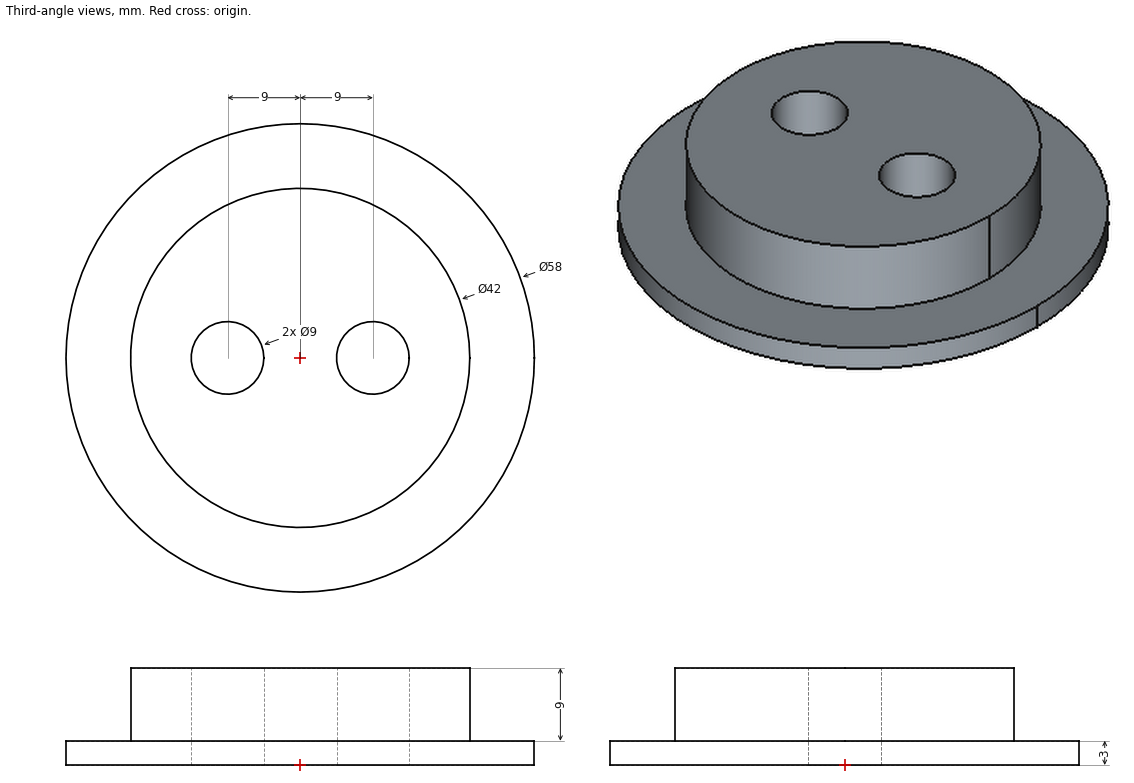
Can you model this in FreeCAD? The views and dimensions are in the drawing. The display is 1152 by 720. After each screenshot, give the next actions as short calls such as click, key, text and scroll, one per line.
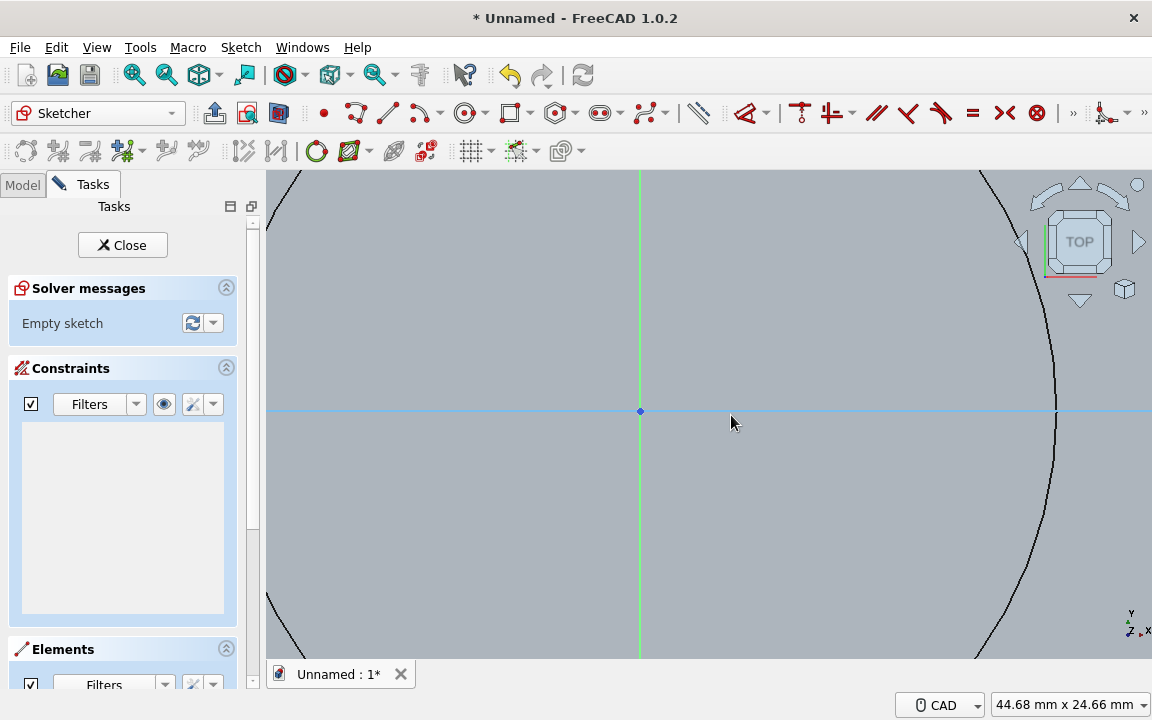
click(466, 114)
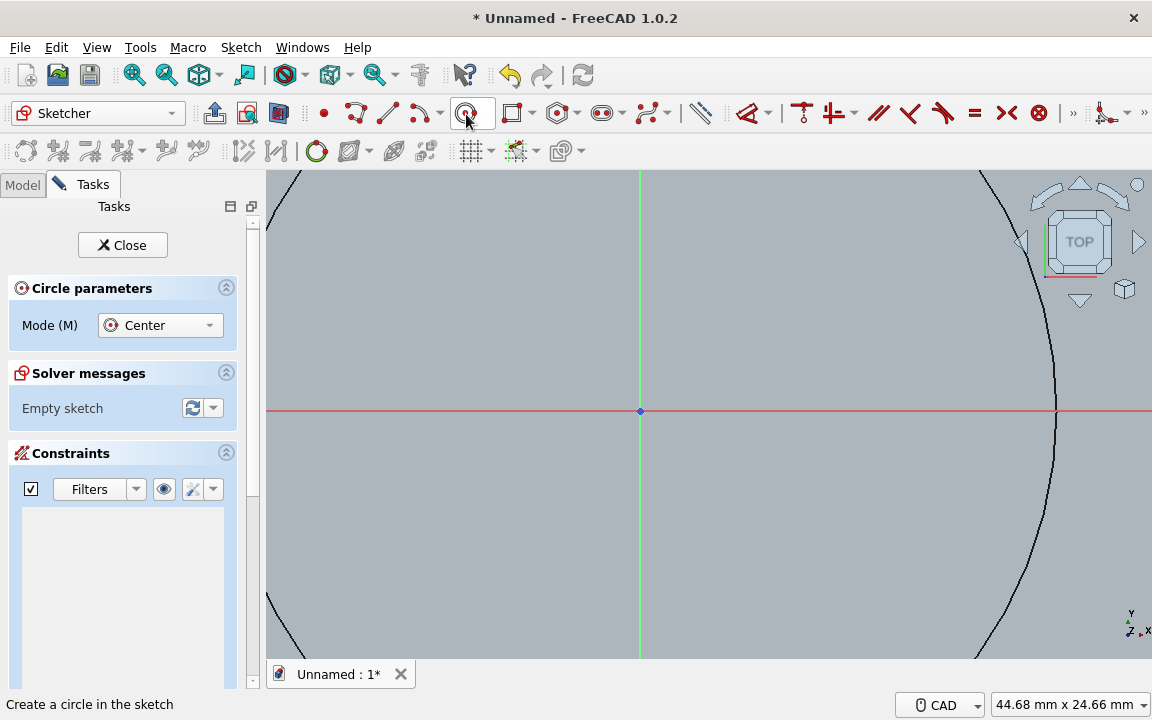
click(462, 411)
move(525, 348)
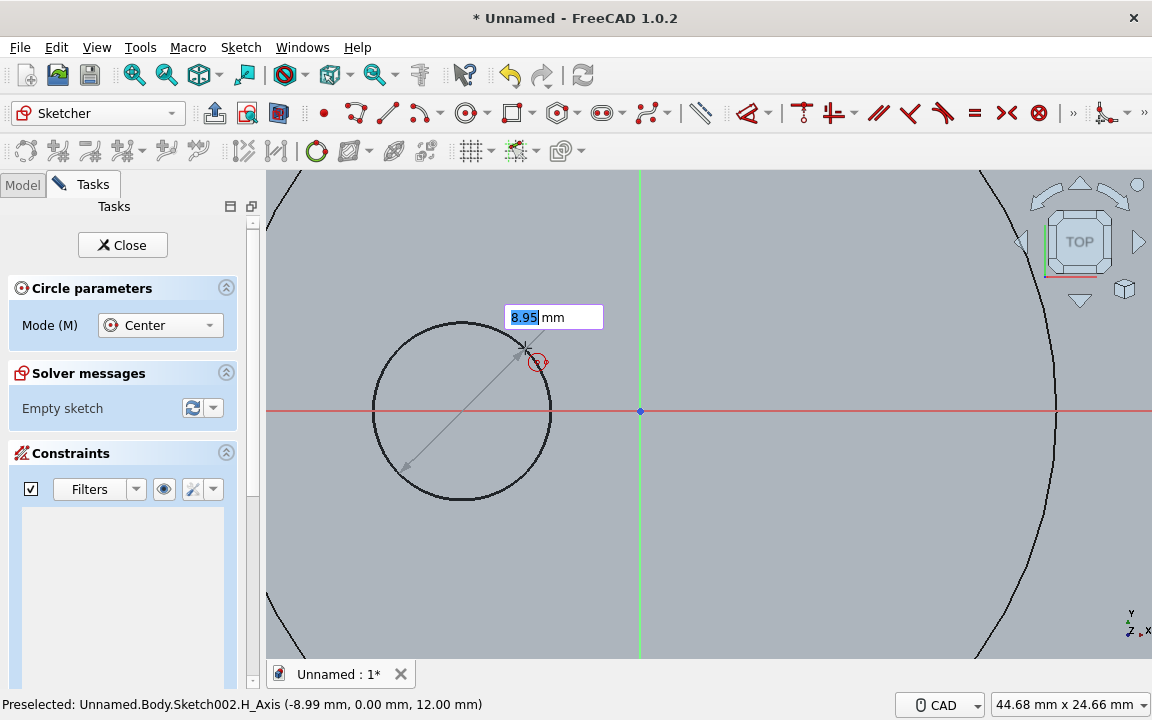
text(9)
key(Return)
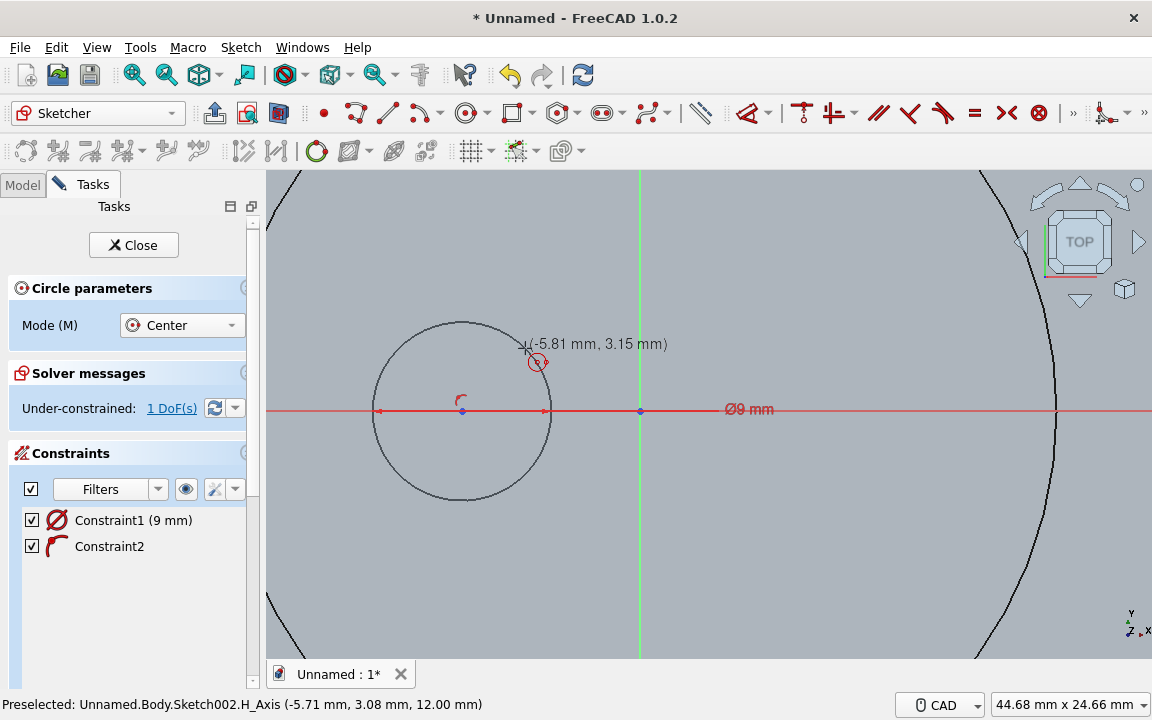
click(819, 411)
move(882, 348)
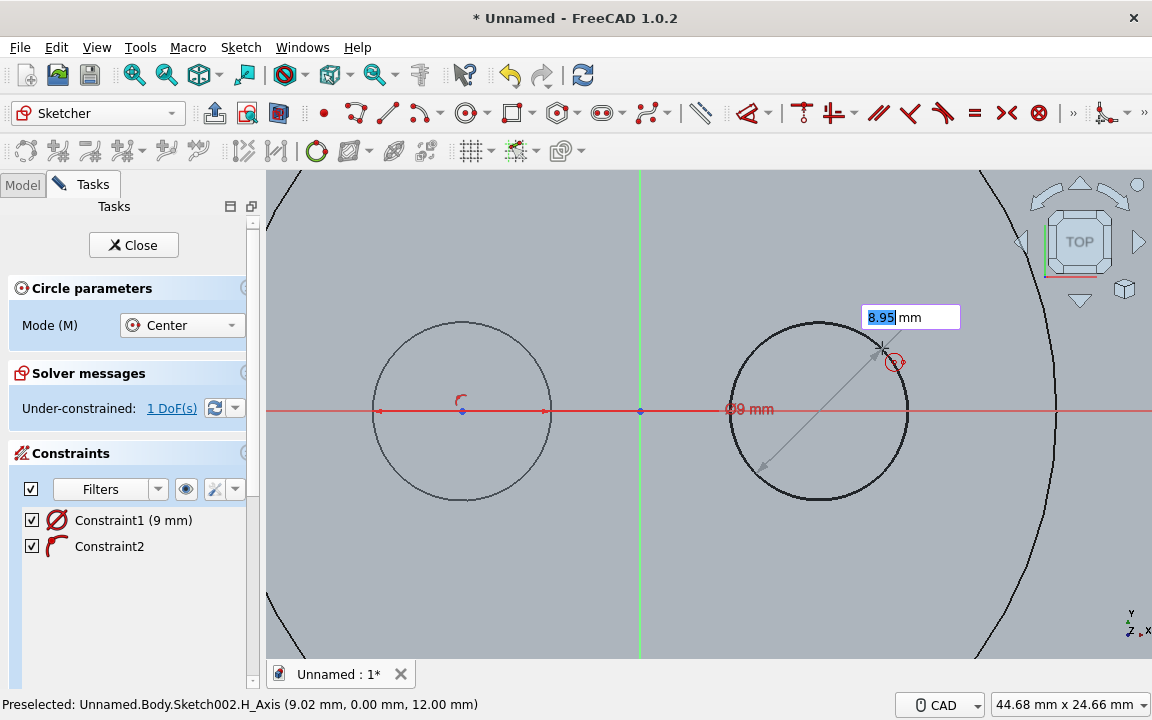
text(9)
key(Return)
key(Escape)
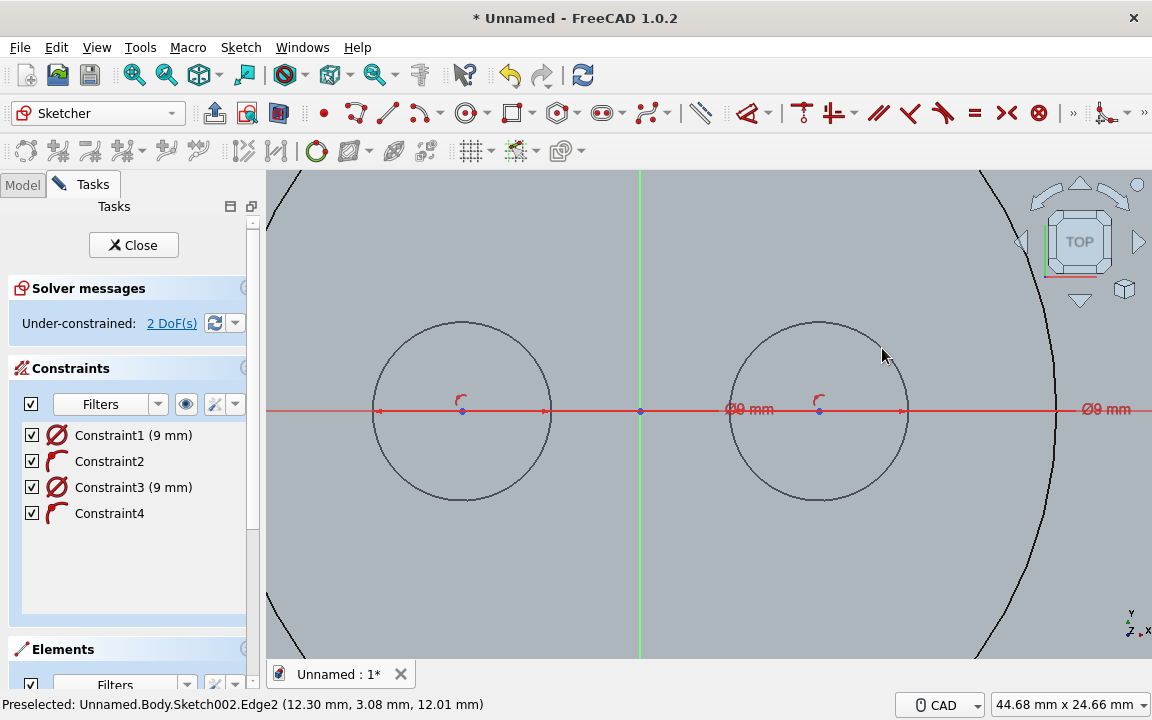
click(748, 114)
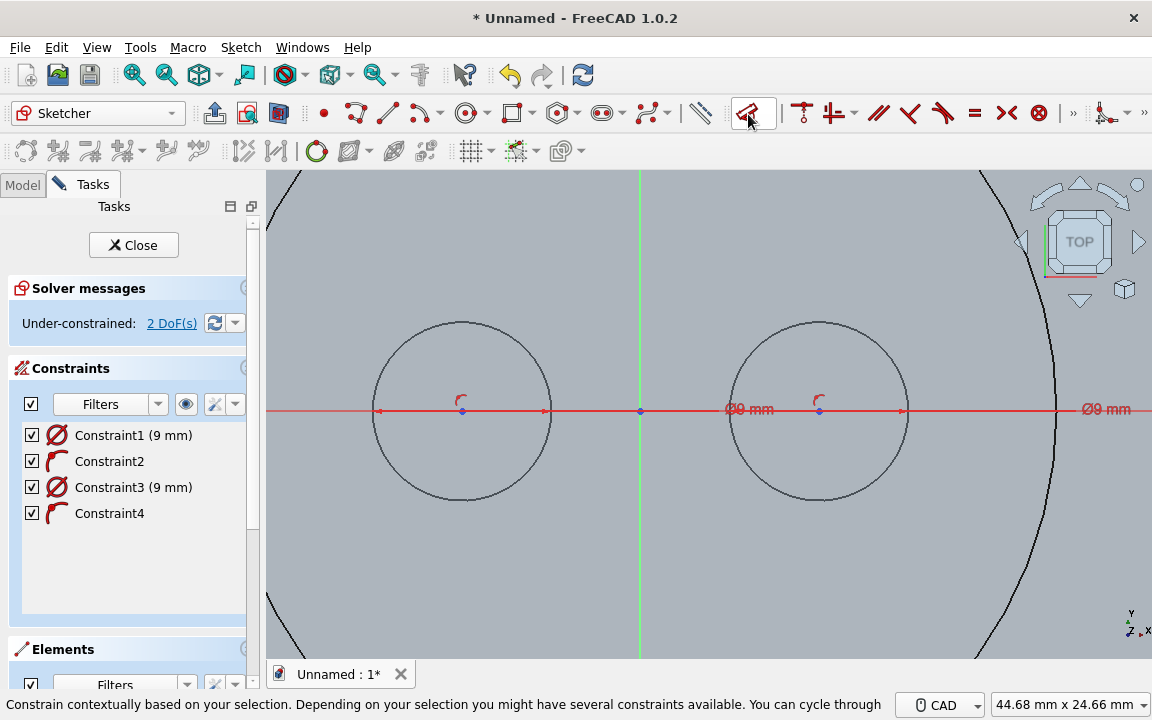
click(462, 411)
click(510, 445)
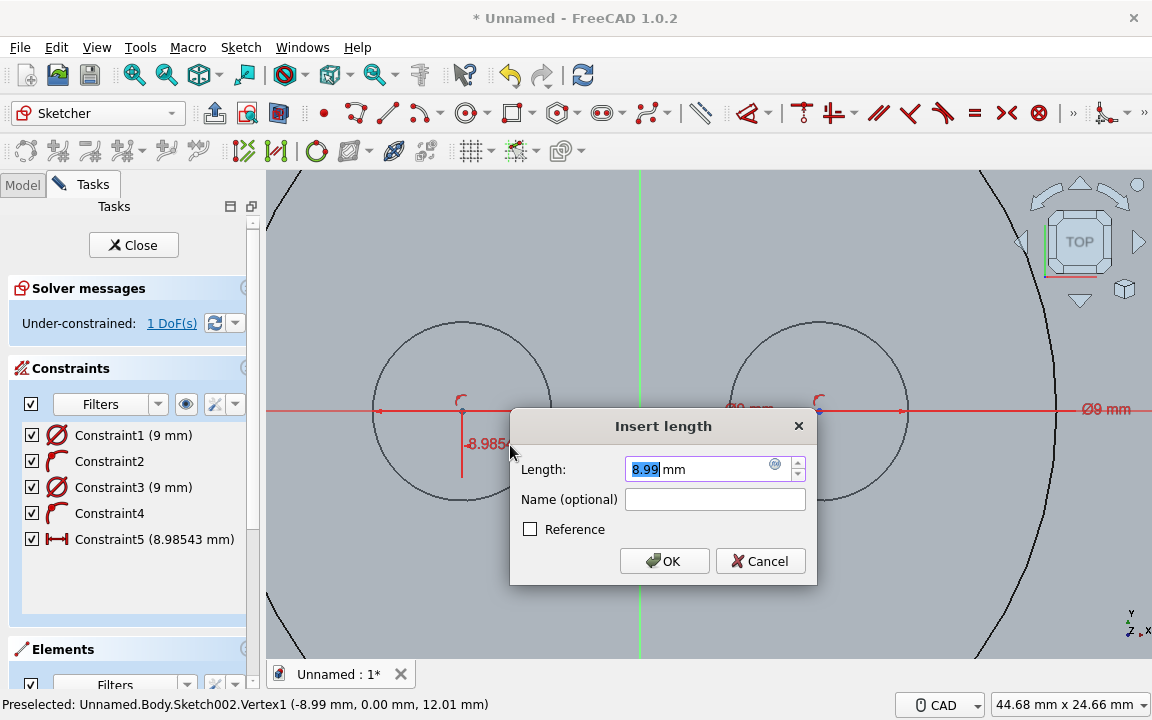
text(9)
key(Return)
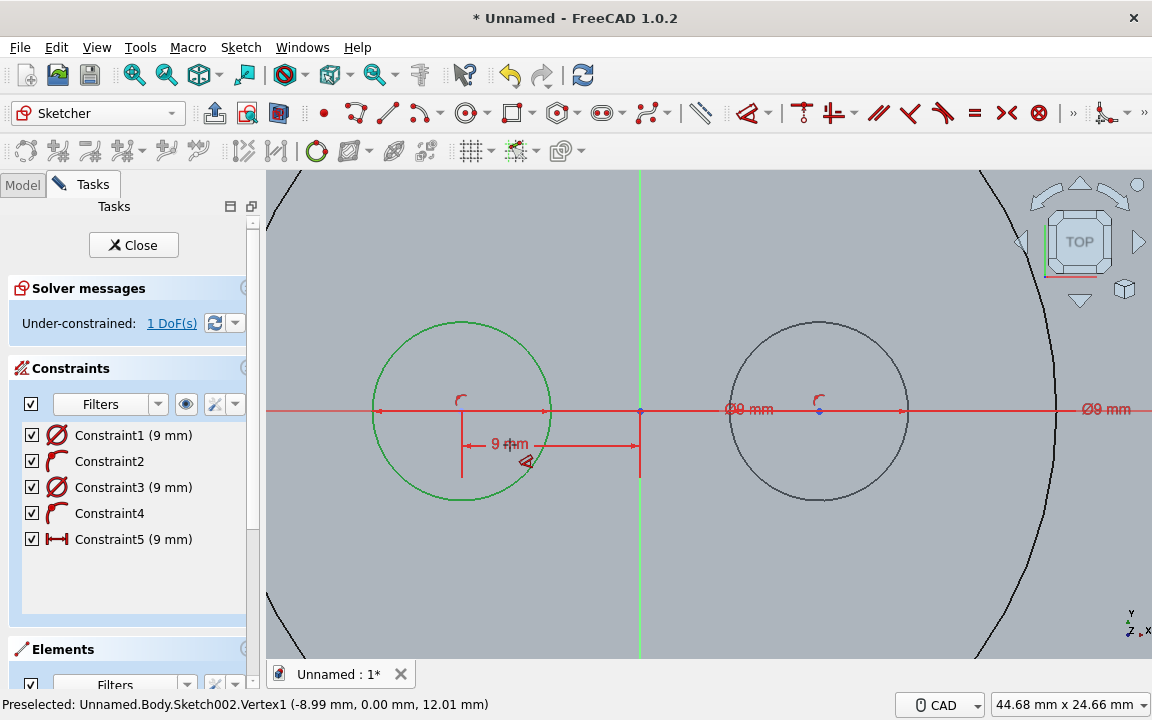
click(819, 411)
click(688, 445)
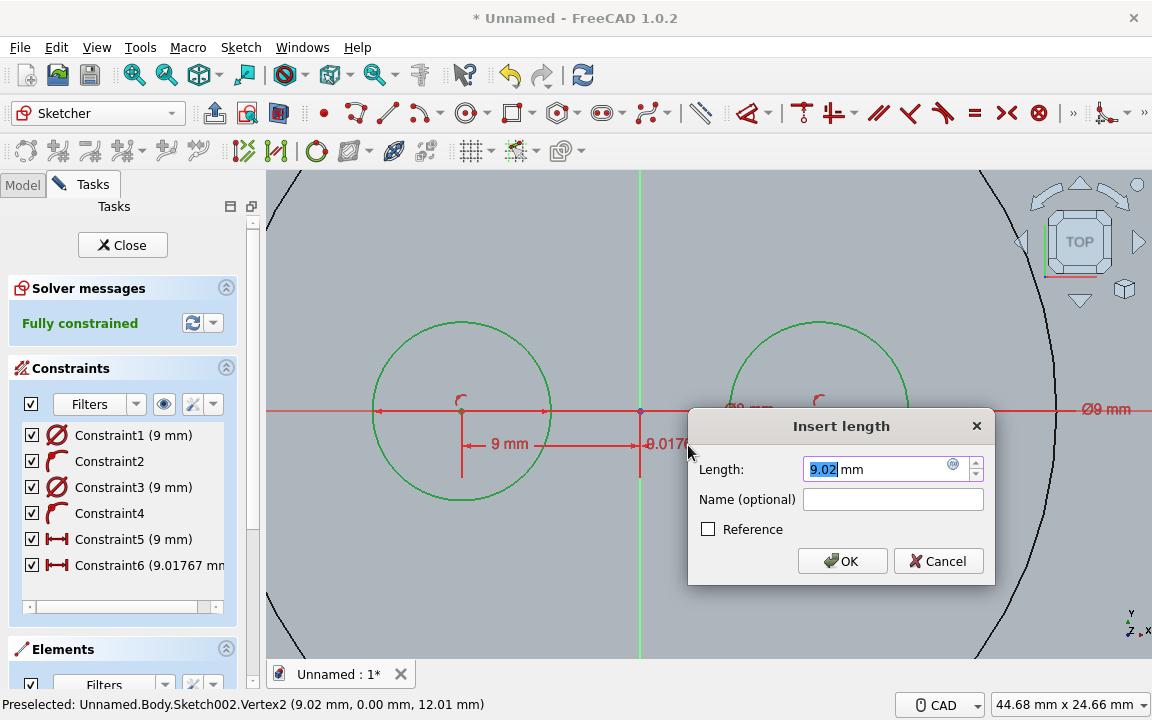
text(9)
key(Return)
key(Escape)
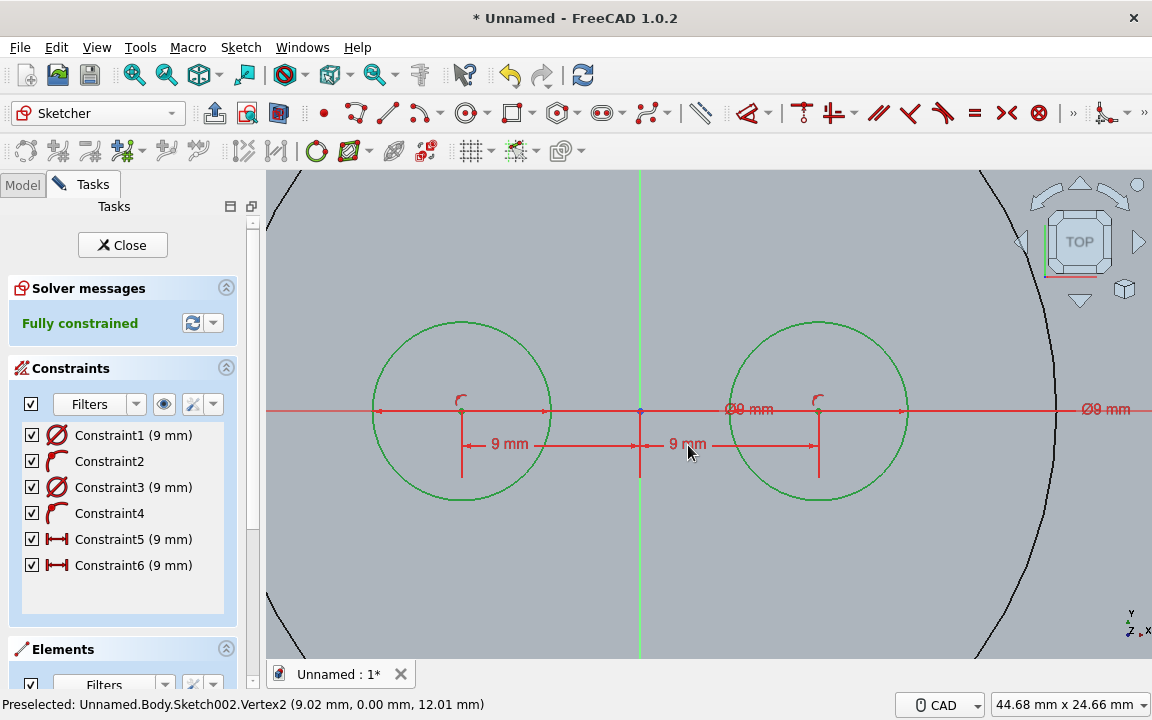
click(123, 245)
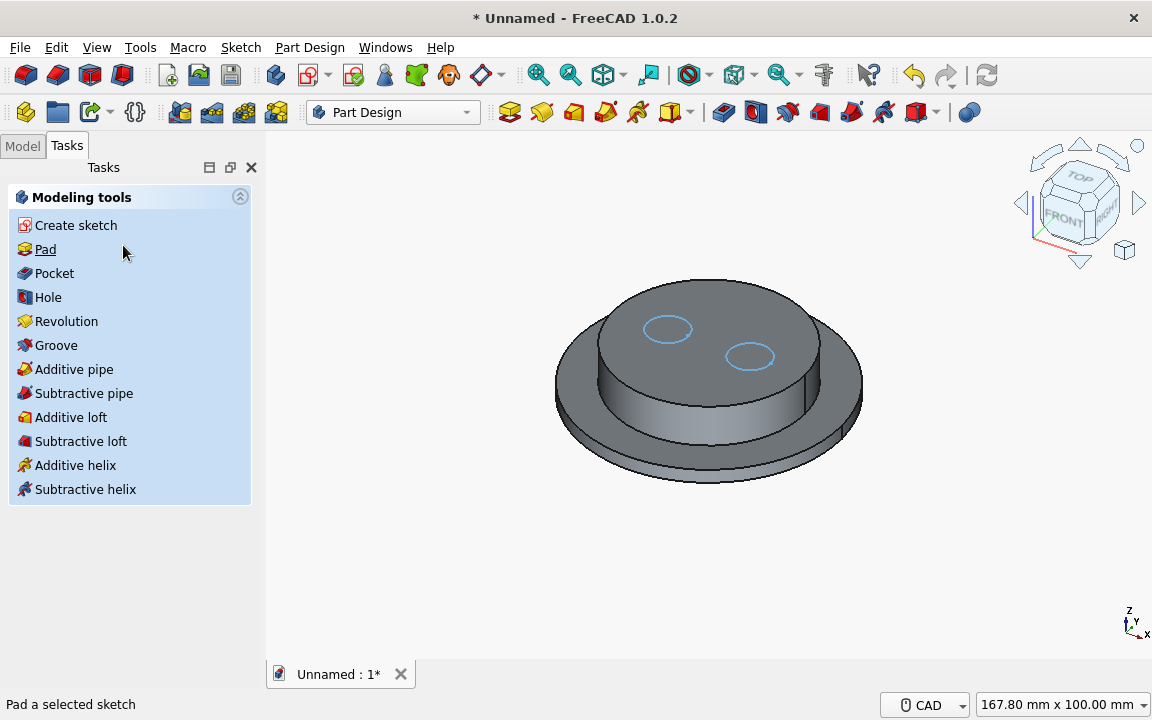
click(724, 112)